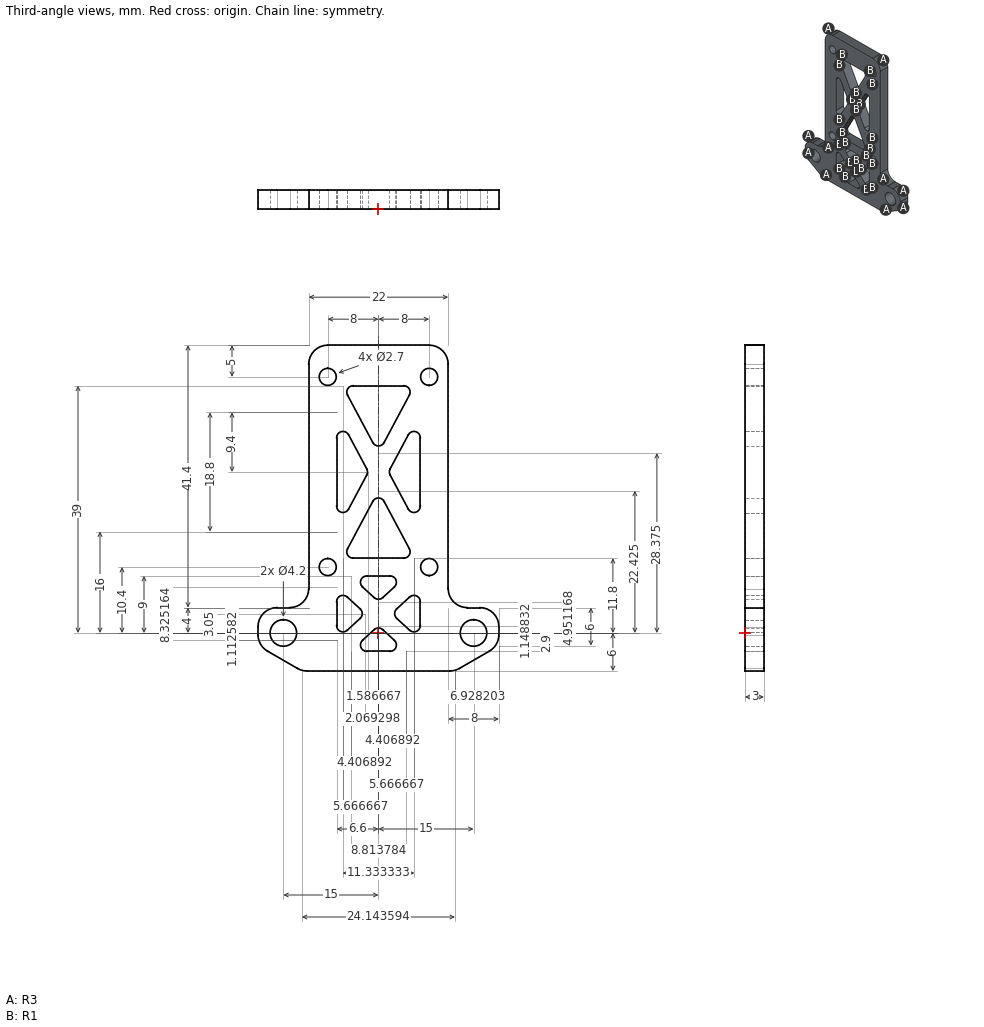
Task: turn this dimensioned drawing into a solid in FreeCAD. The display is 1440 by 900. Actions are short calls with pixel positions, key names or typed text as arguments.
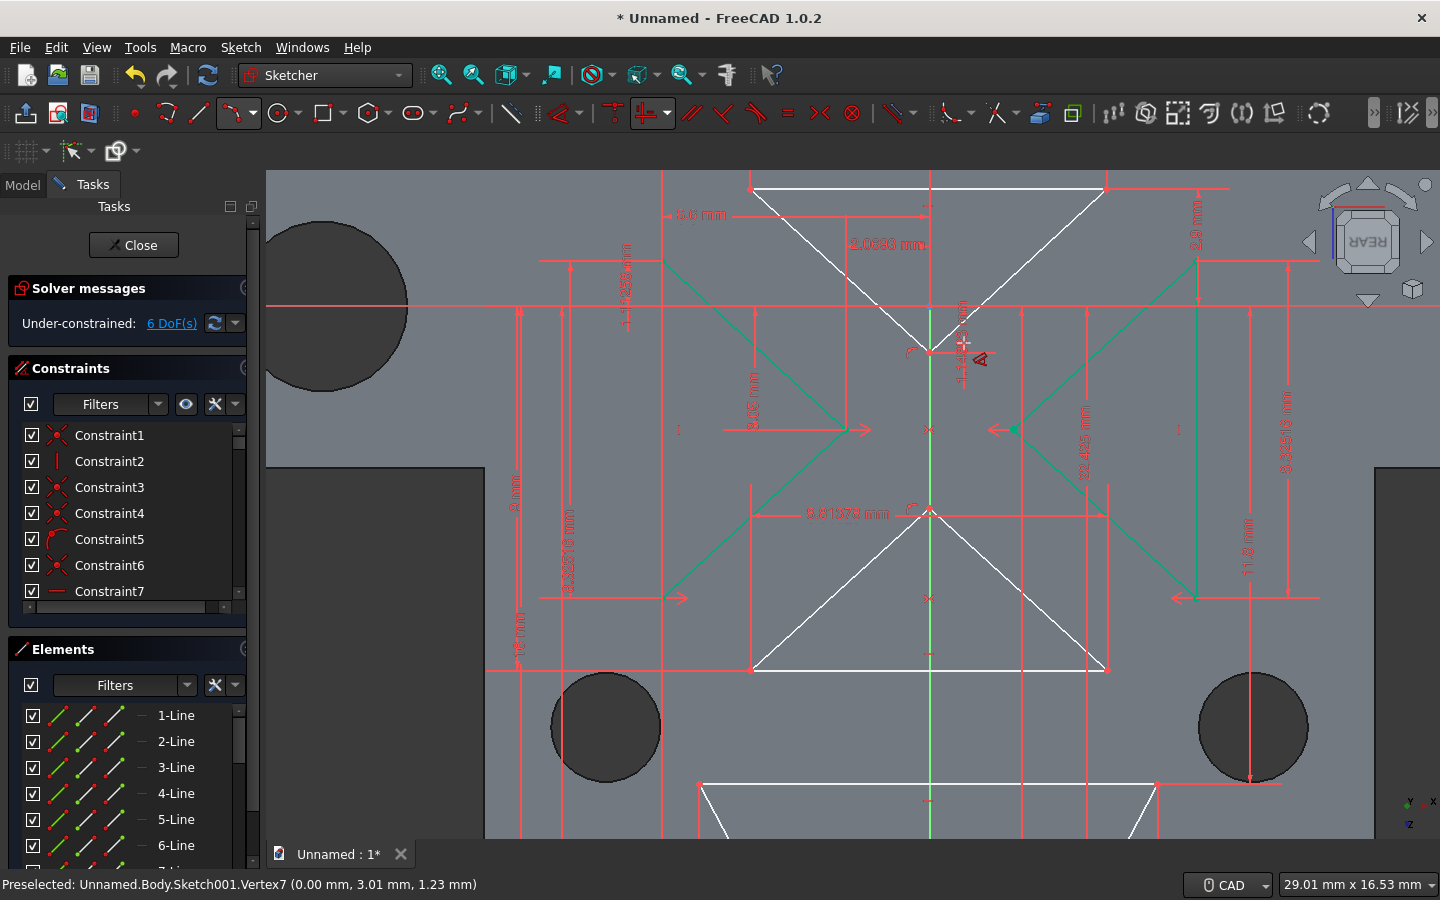
scroll(737, 330, down, 7)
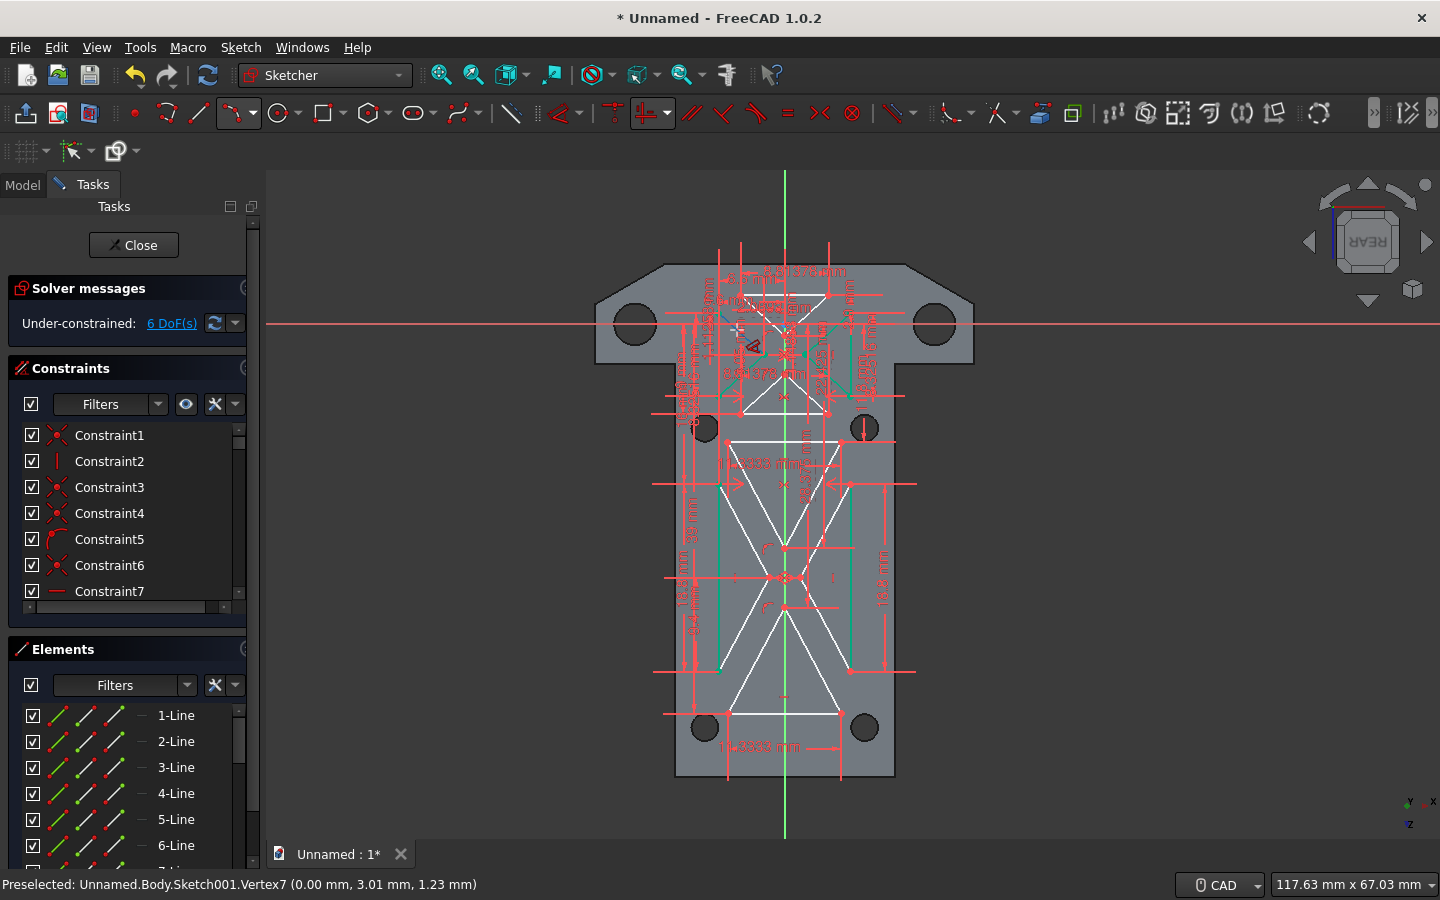
click(829, 295)
click(807, 237)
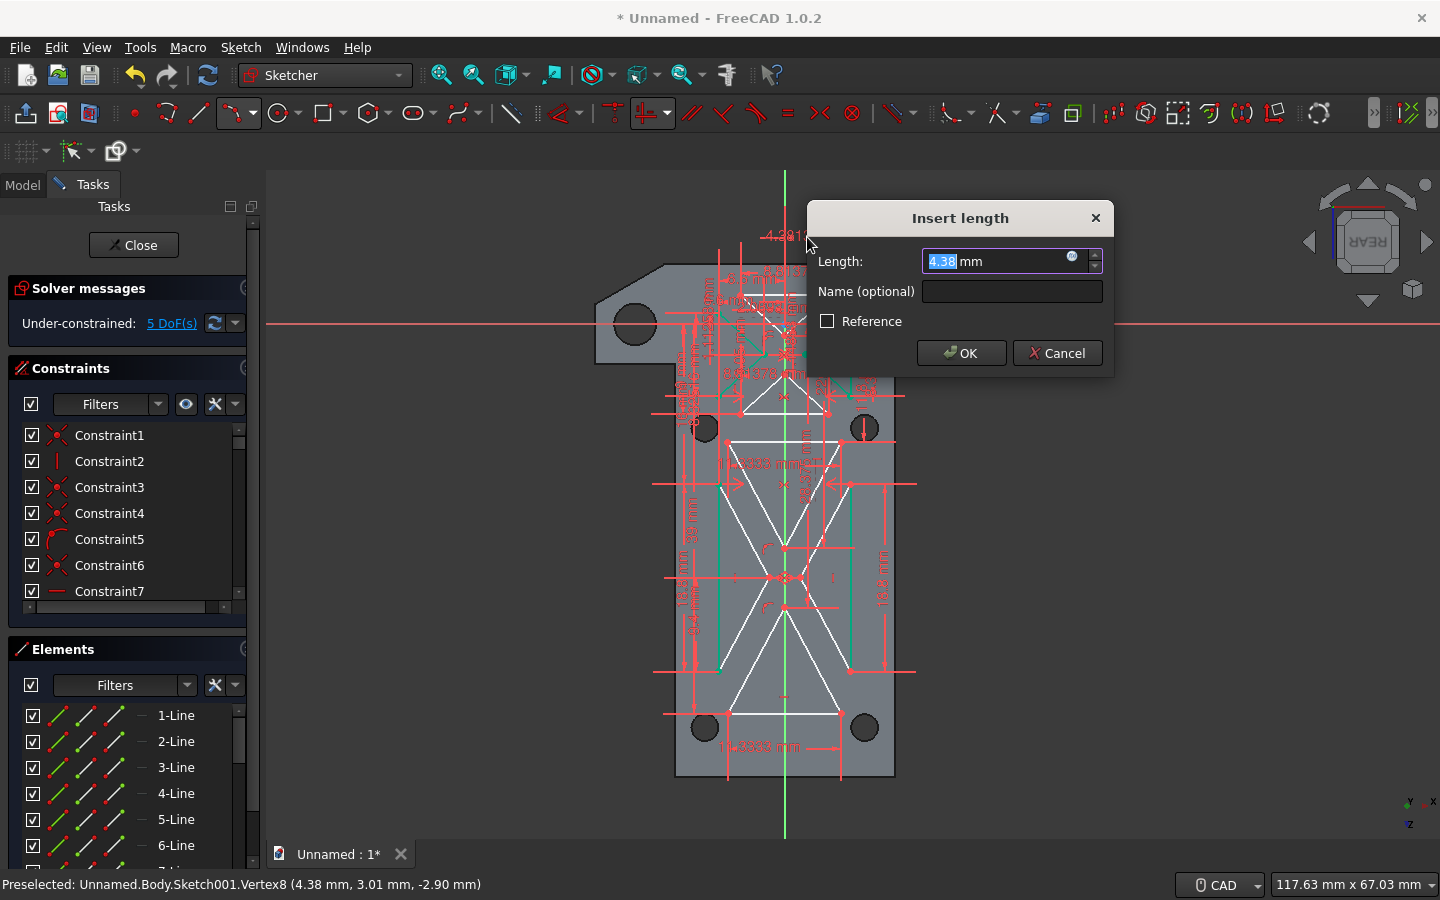
text(4.406892)
key(Return)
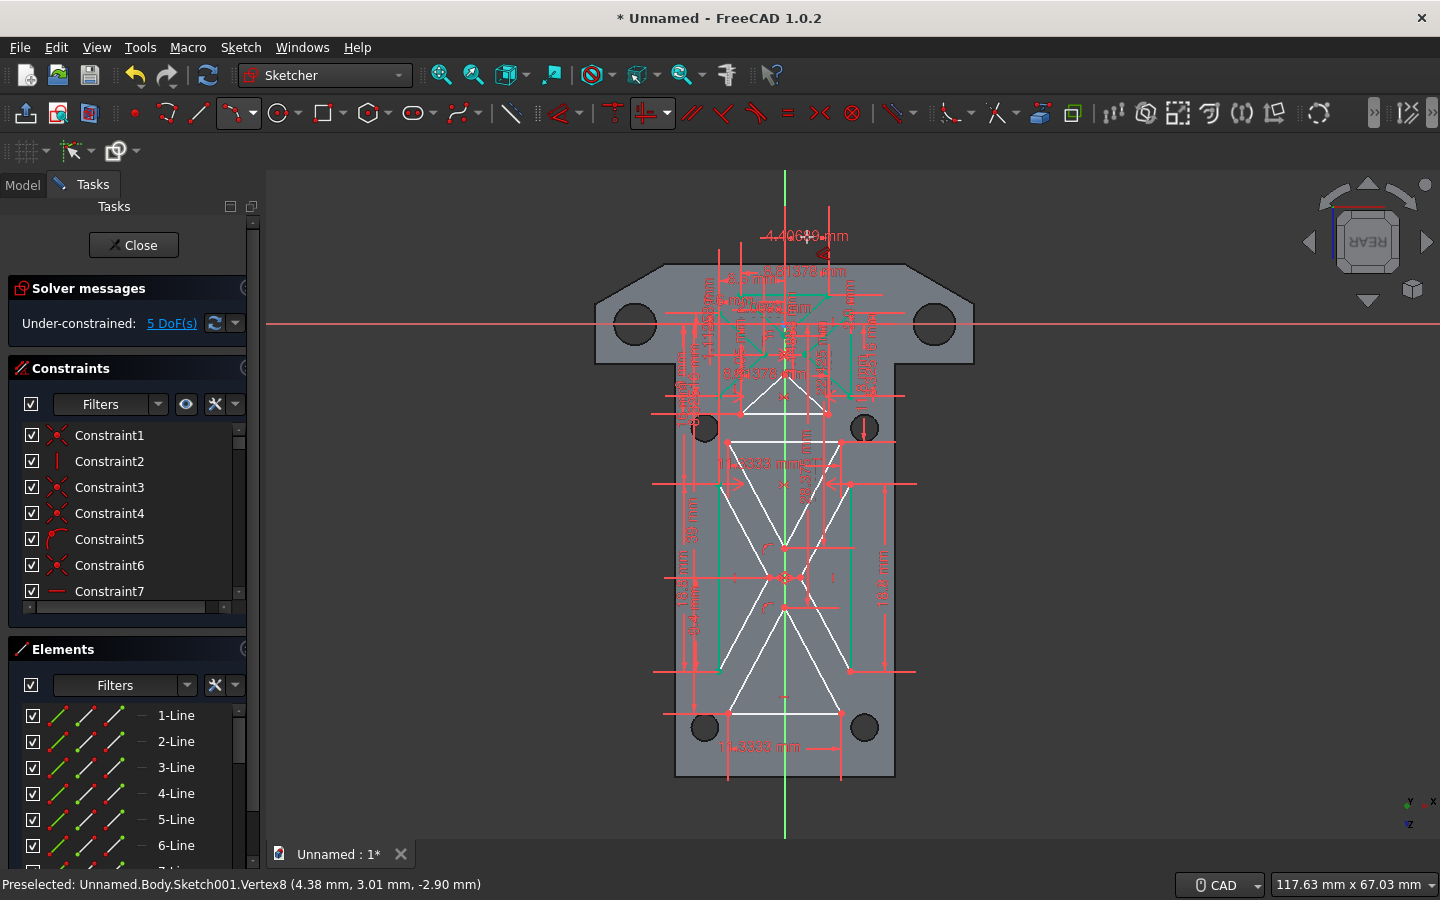
click(785, 374)
click(655, 349)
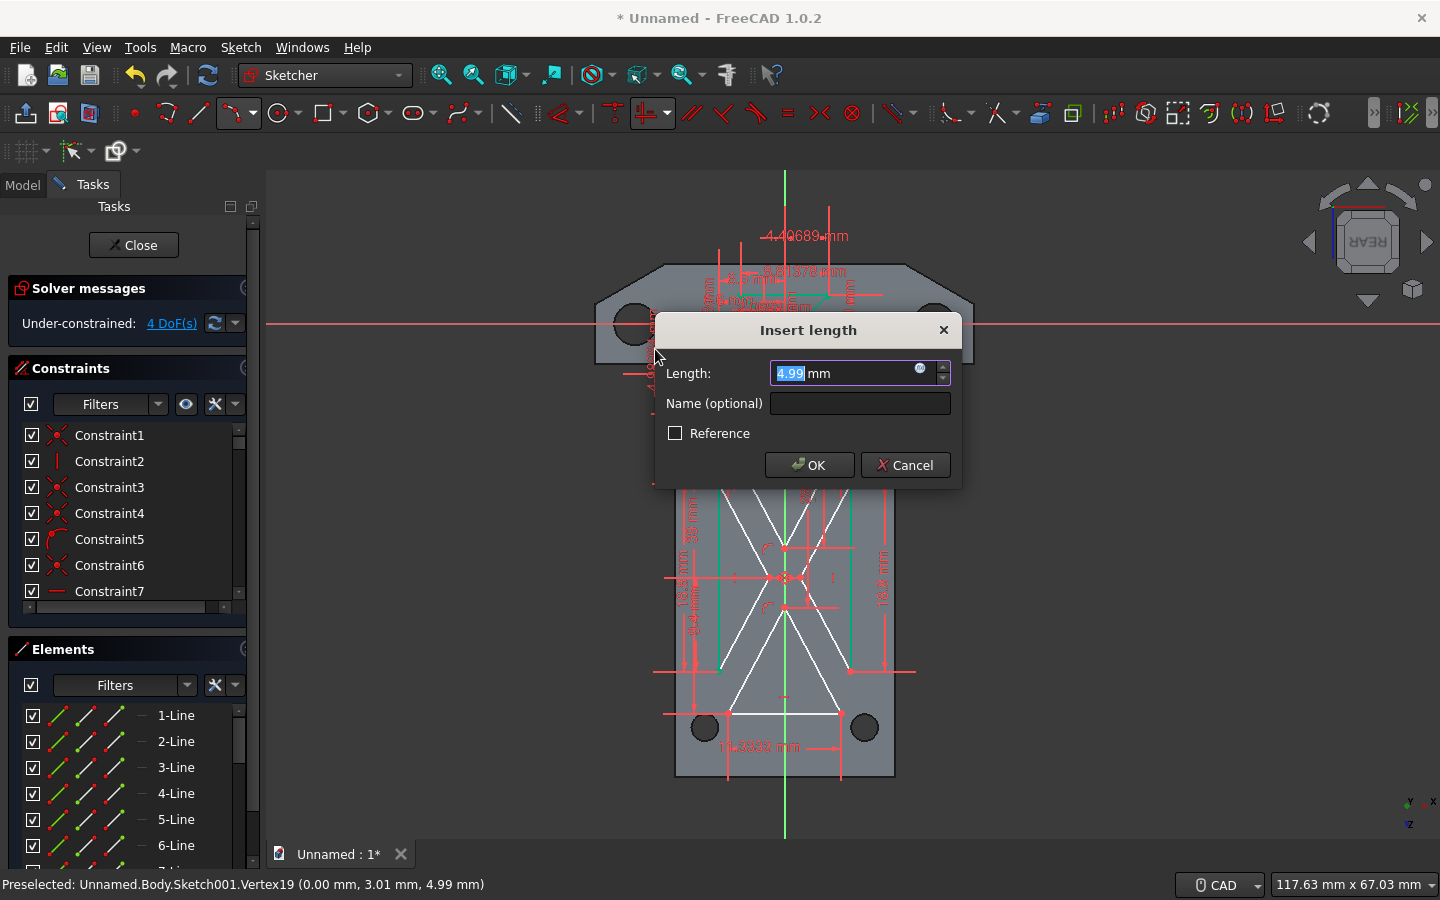
text(4.951168)
key(Return)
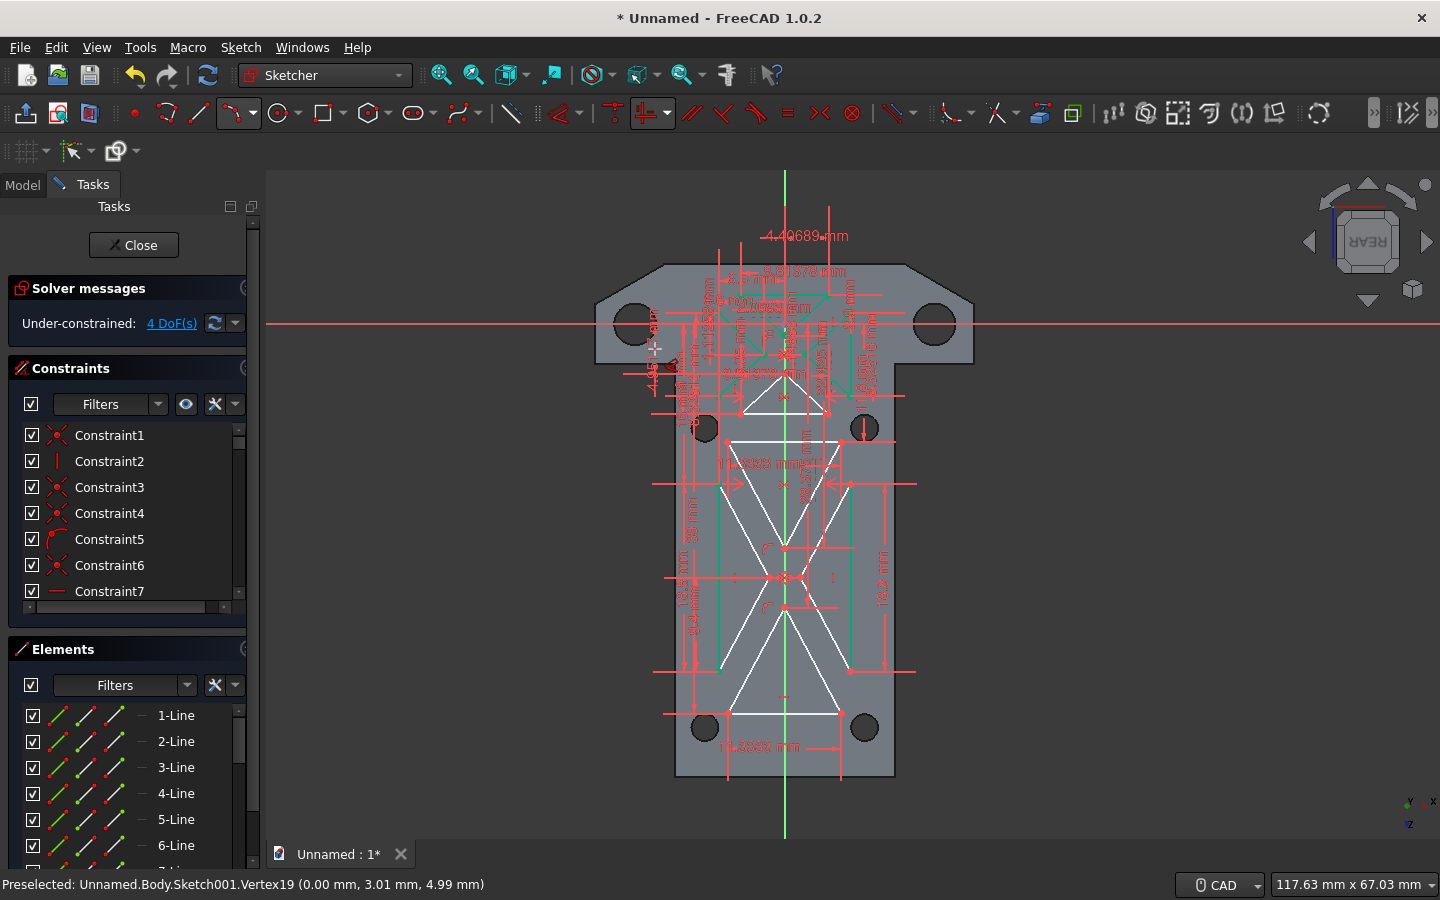
click(741, 414)
click(763, 266)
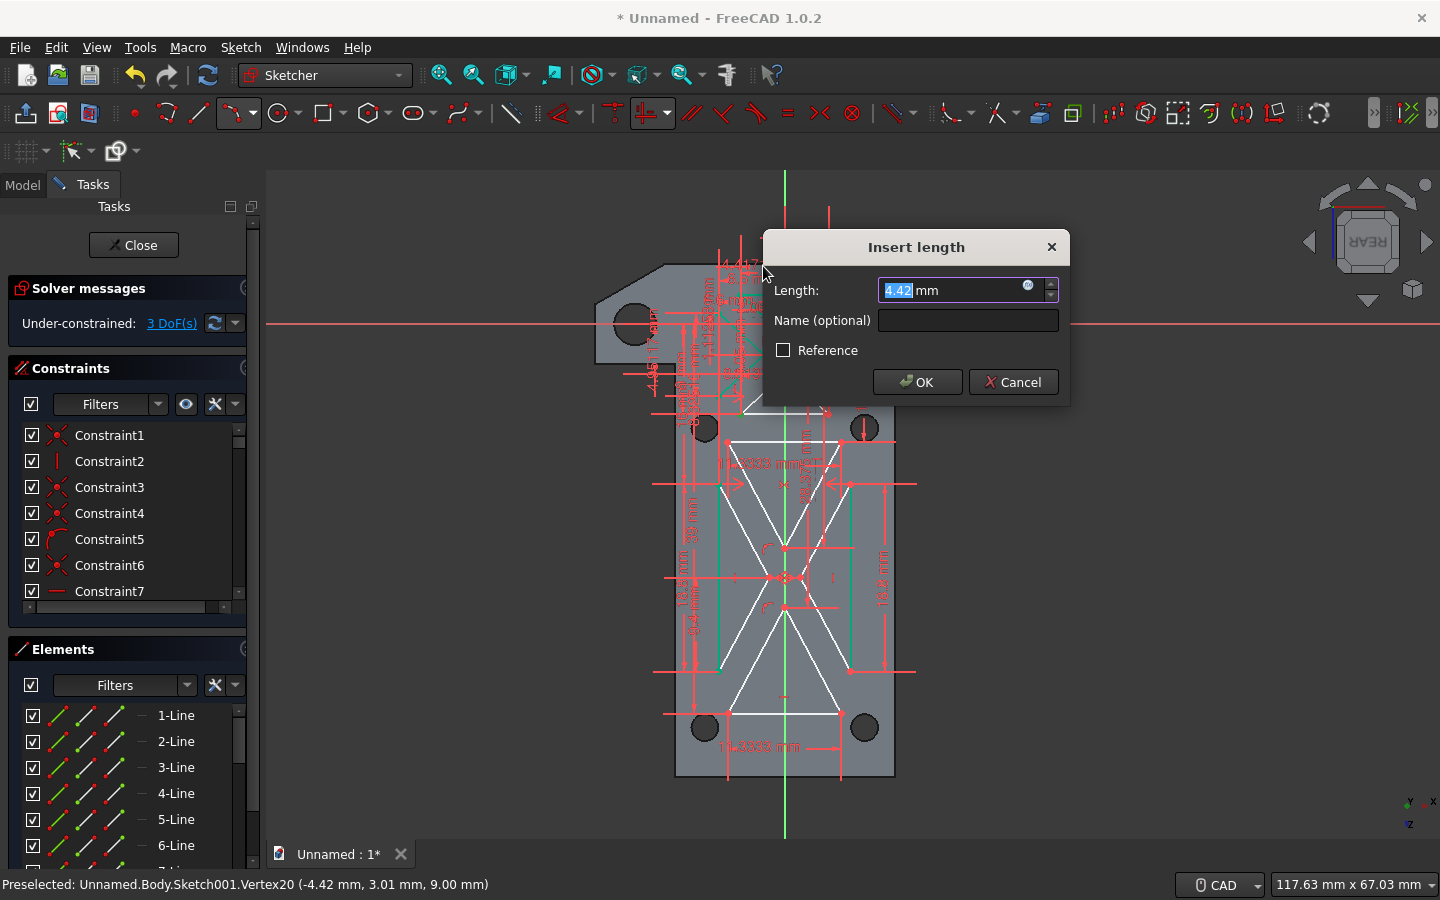
text(4.406892)
key(Return)